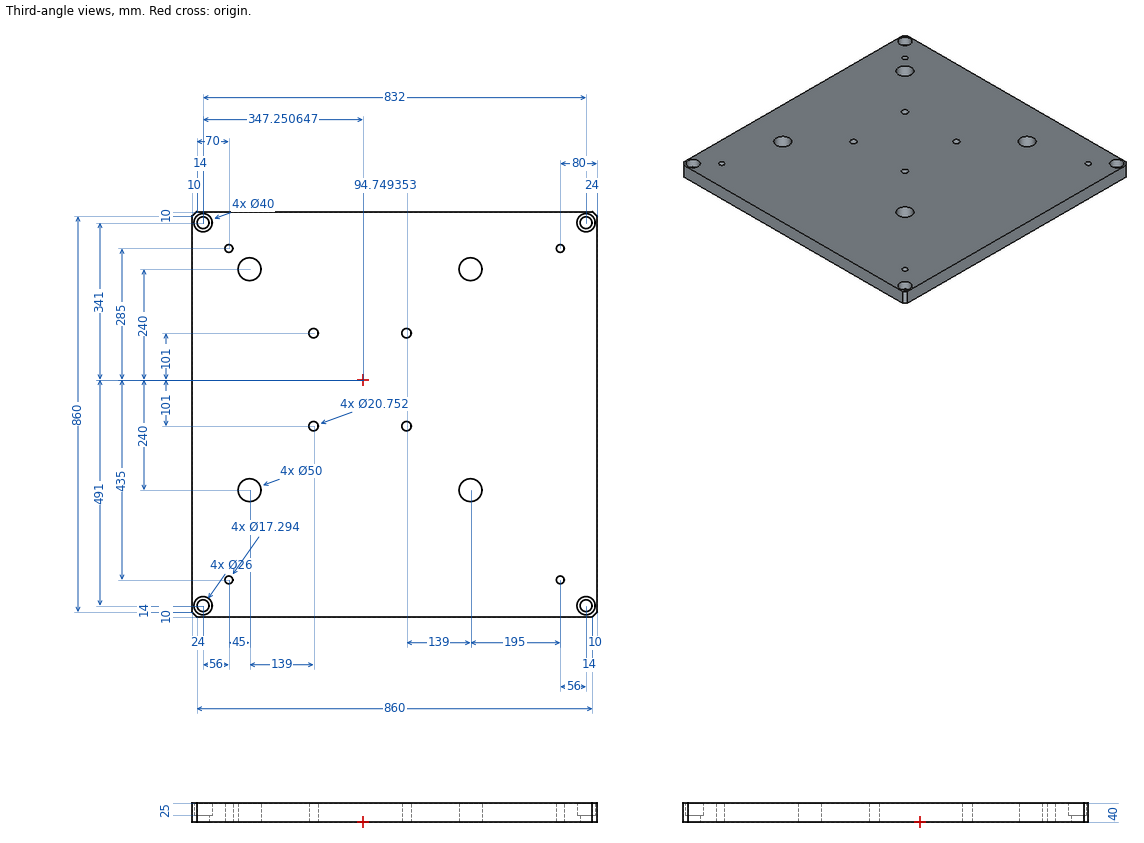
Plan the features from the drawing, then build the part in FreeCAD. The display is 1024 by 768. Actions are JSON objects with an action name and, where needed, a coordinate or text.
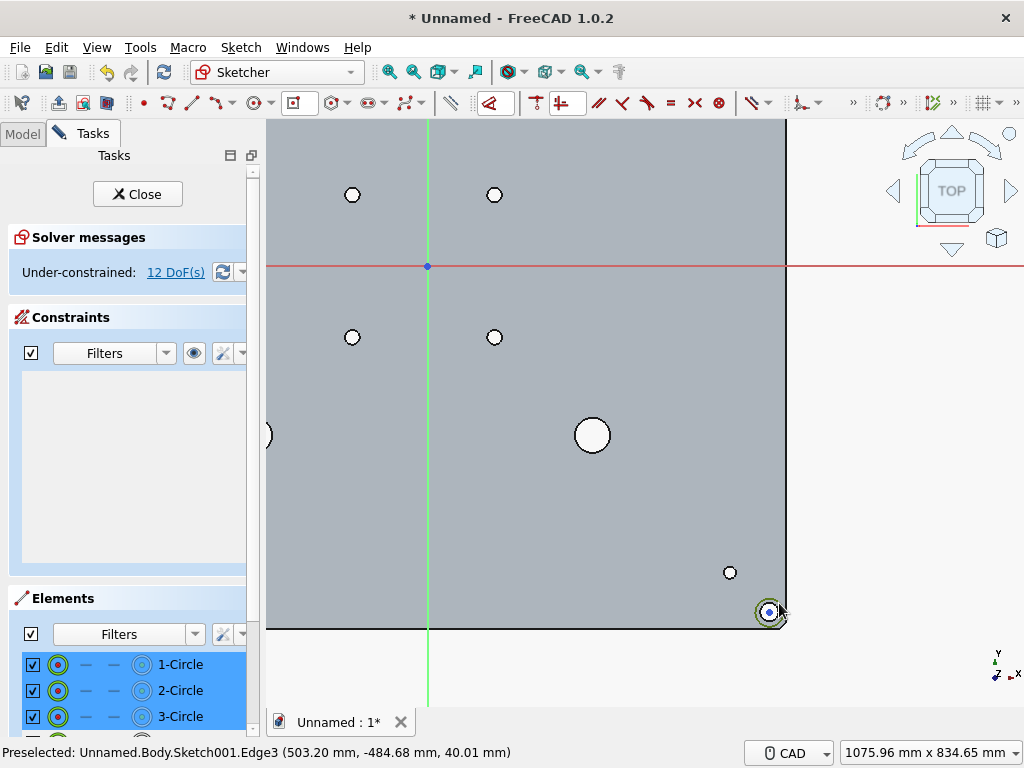
{"action": "scroll", "coordinate": [780, 604], "scroll_direction": "down", "scroll_amount": 2}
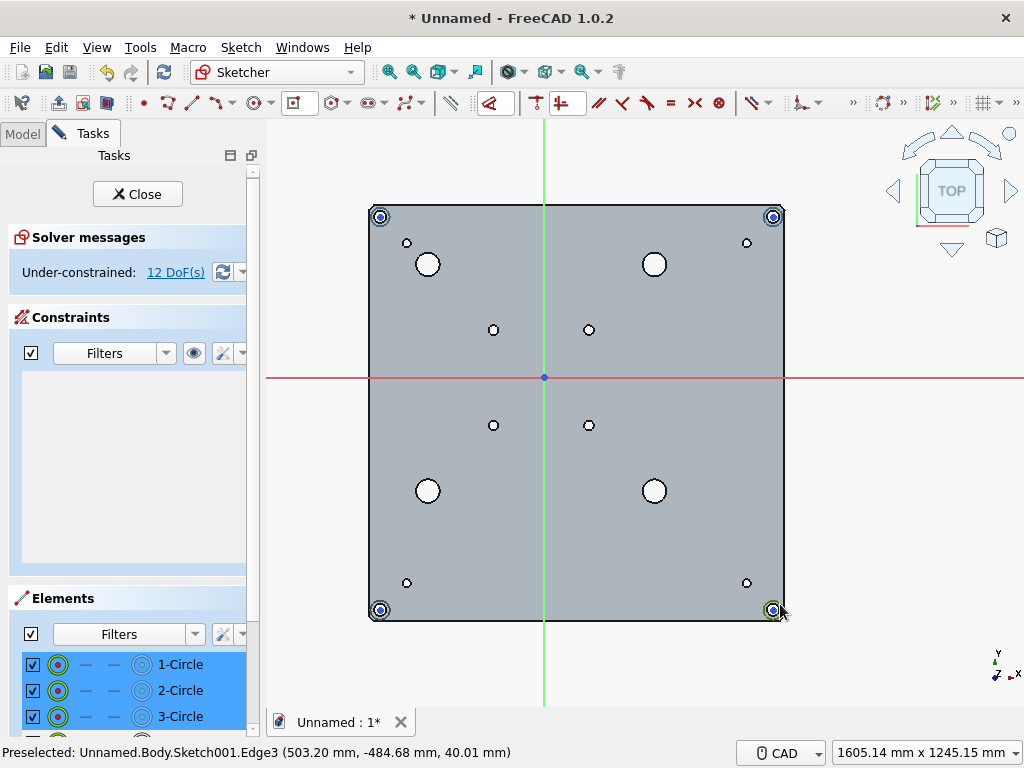
{"action": "scroll", "coordinate": [387, 603], "scroll_direction": "up", "scroll_amount": 2}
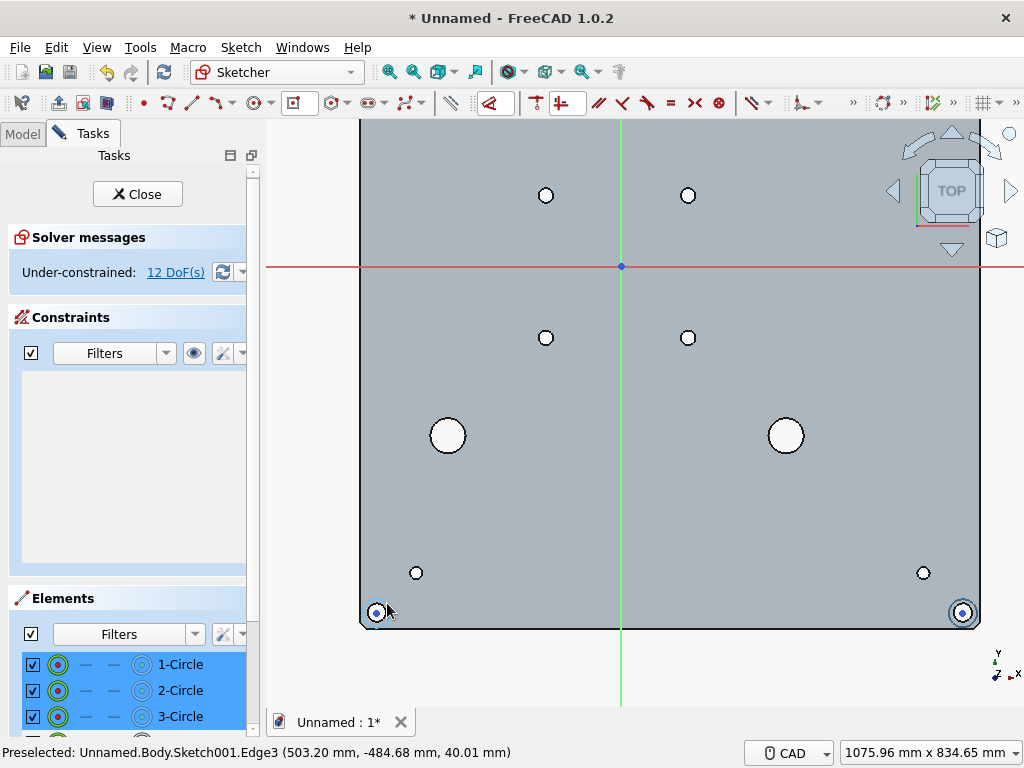
{"action": "left_click", "coordinate": [387, 603]}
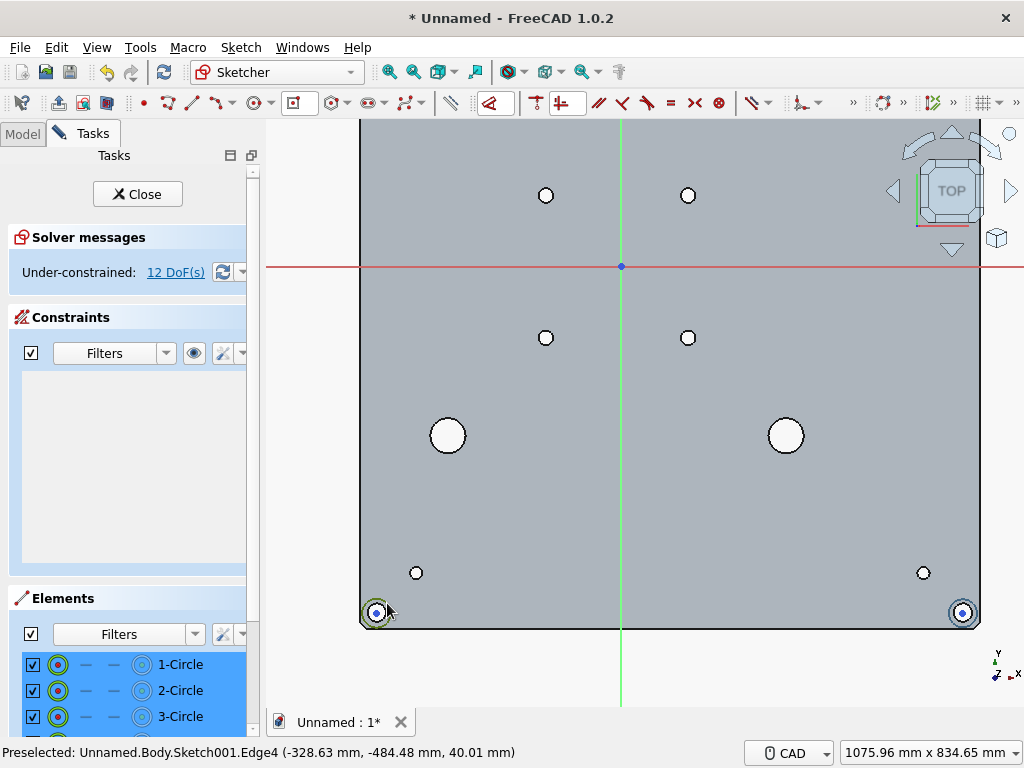
{"action": "left_click", "coordinate": [672, 104]}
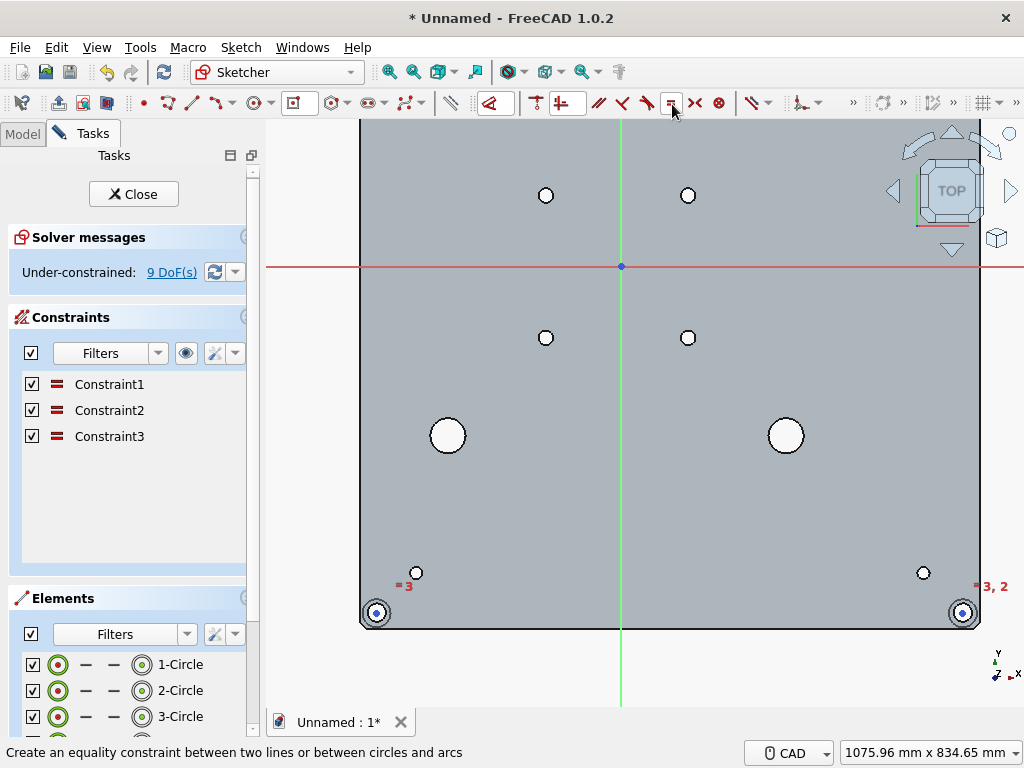
{"action": "scroll", "coordinate": [387, 603], "scroll_direction": "down", "scroll_amount": 2}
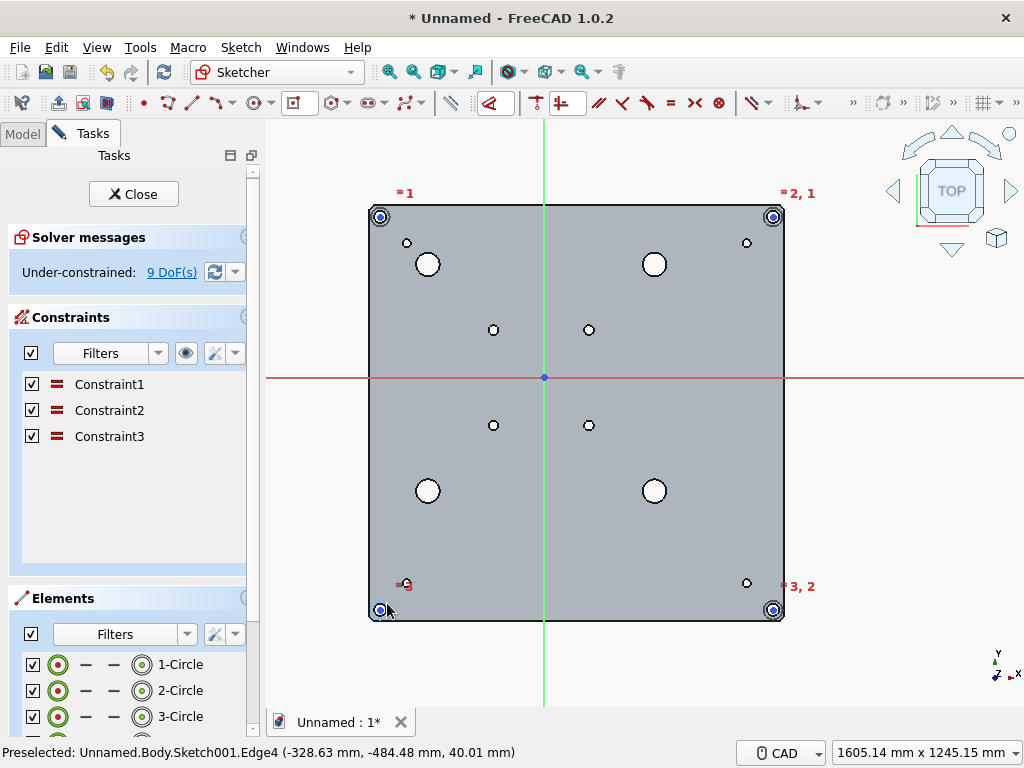
{"action": "left_click", "coordinate": [380, 217]}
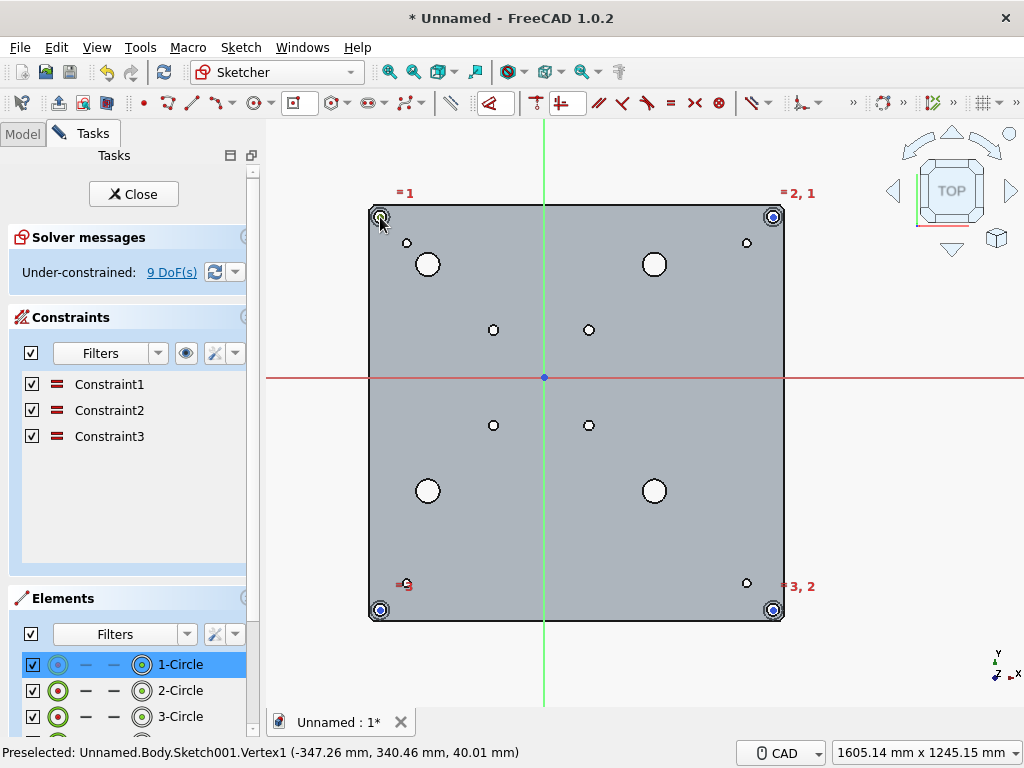
{"action": "left_click", "coordinate": [773, 217]}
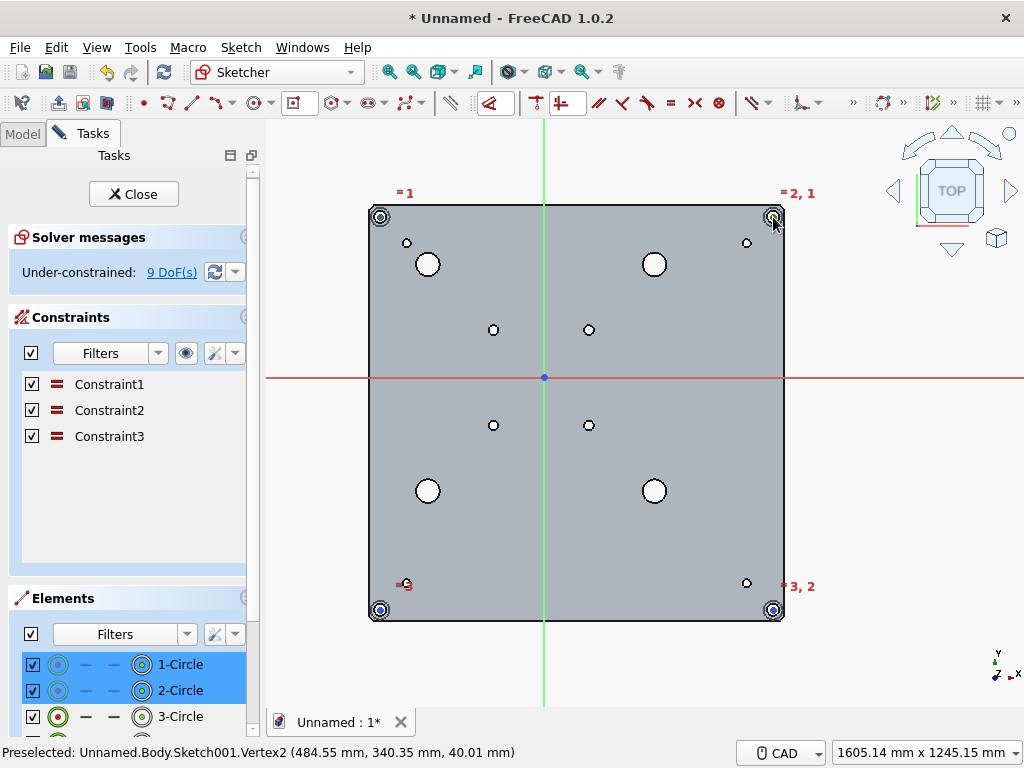
{"action": "key", "text": "h"}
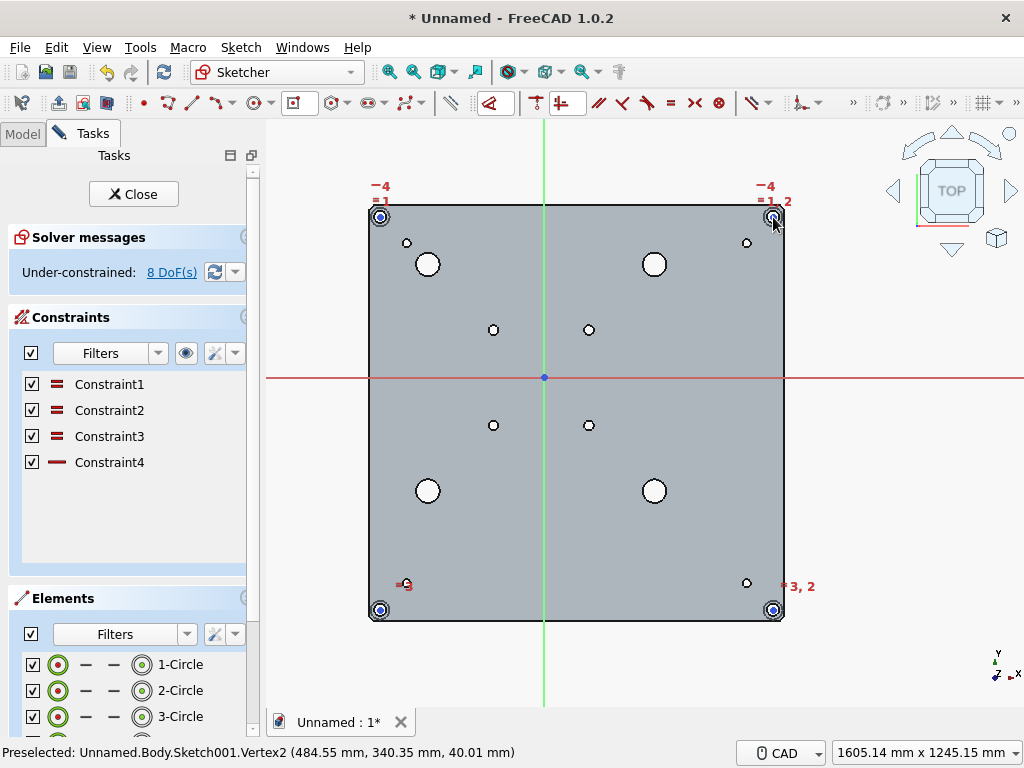
{"action": "left_click", "coordinate": [773, 217]}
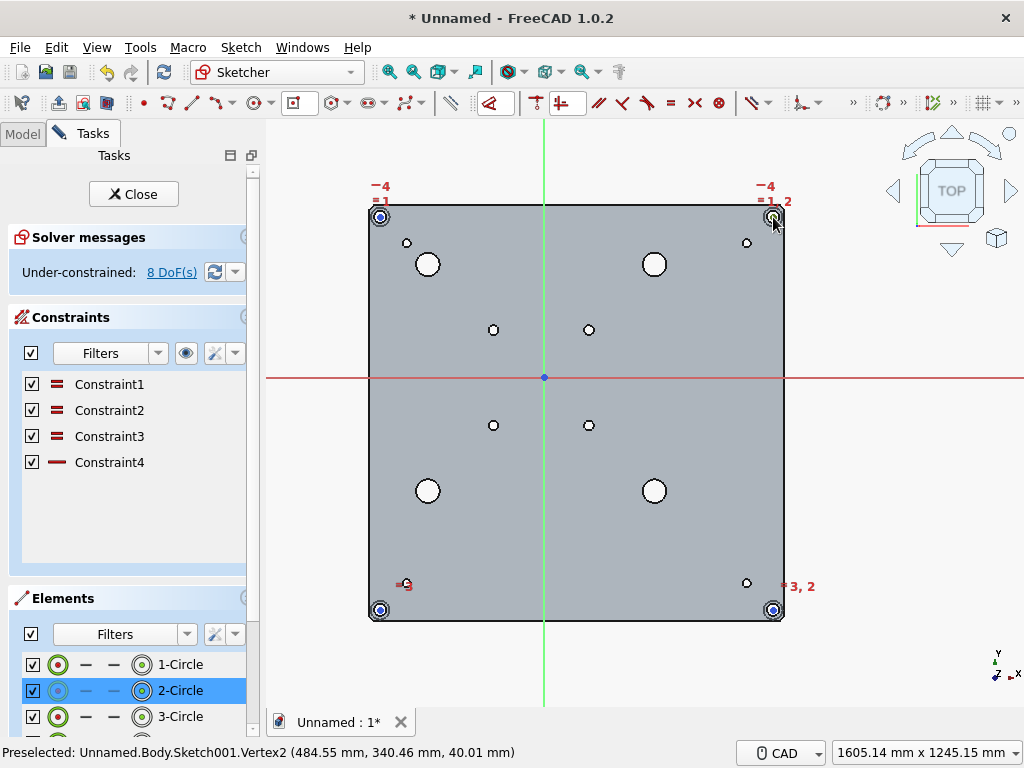
{"action": "left_click", "coordinate": [773, 610]}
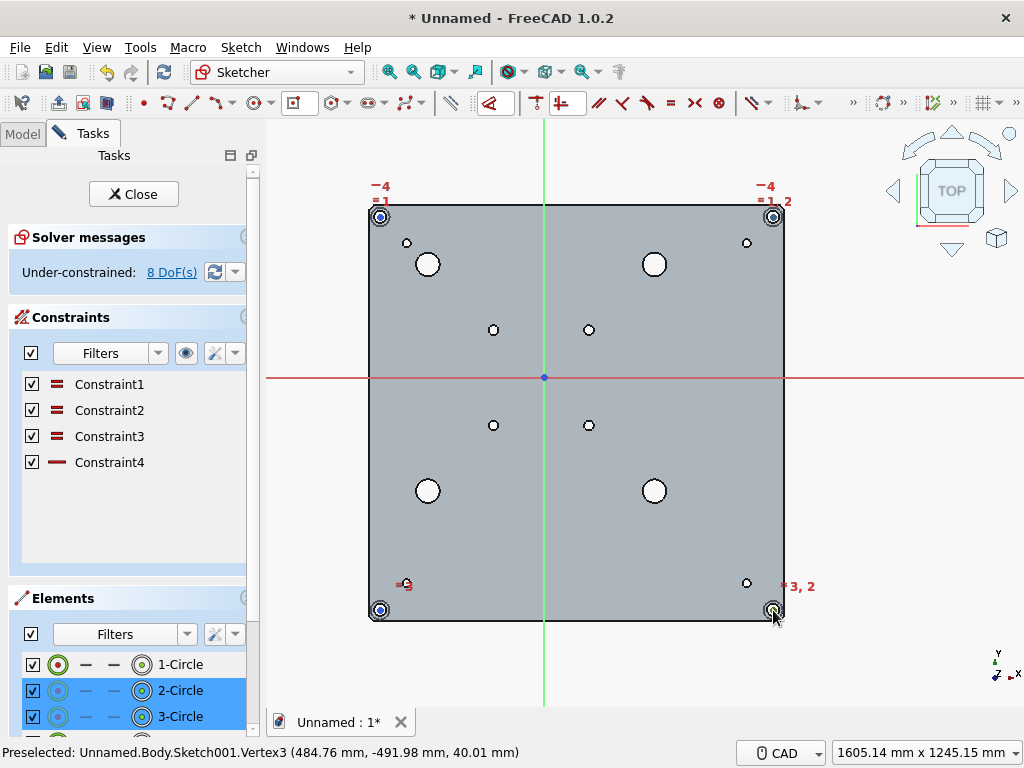
{"action": "key", "text": "v"}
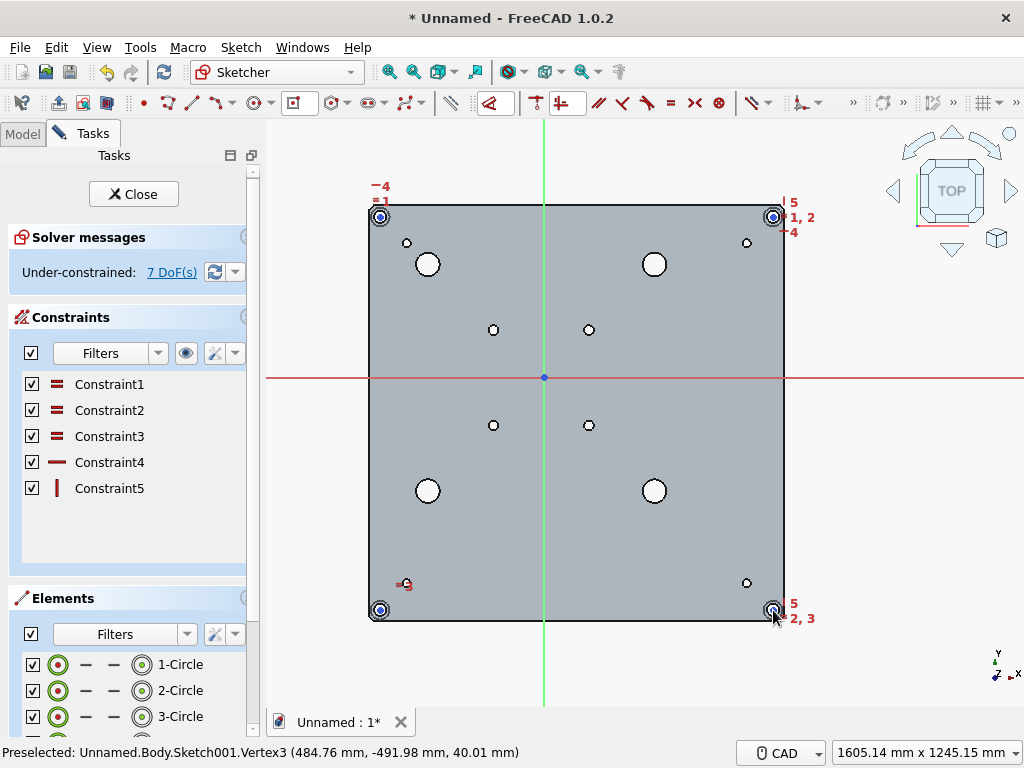
{"action": "left_click", "coordinate": [380, 217]}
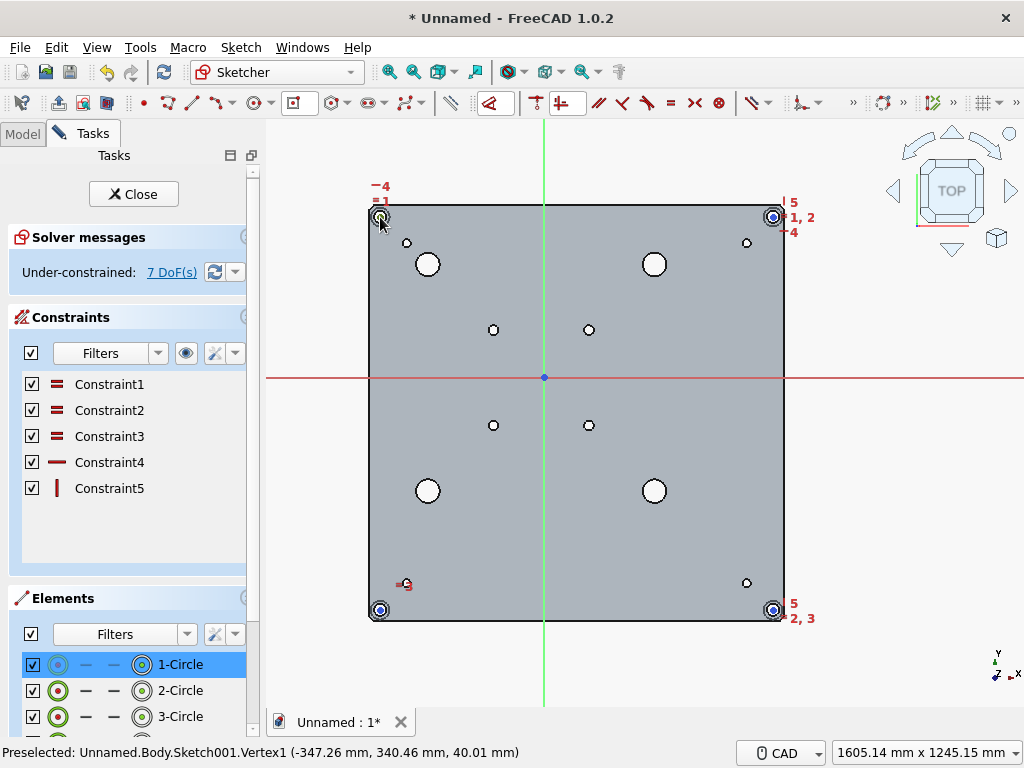
{"action": "left_click", "coordinate": [380, 610]}